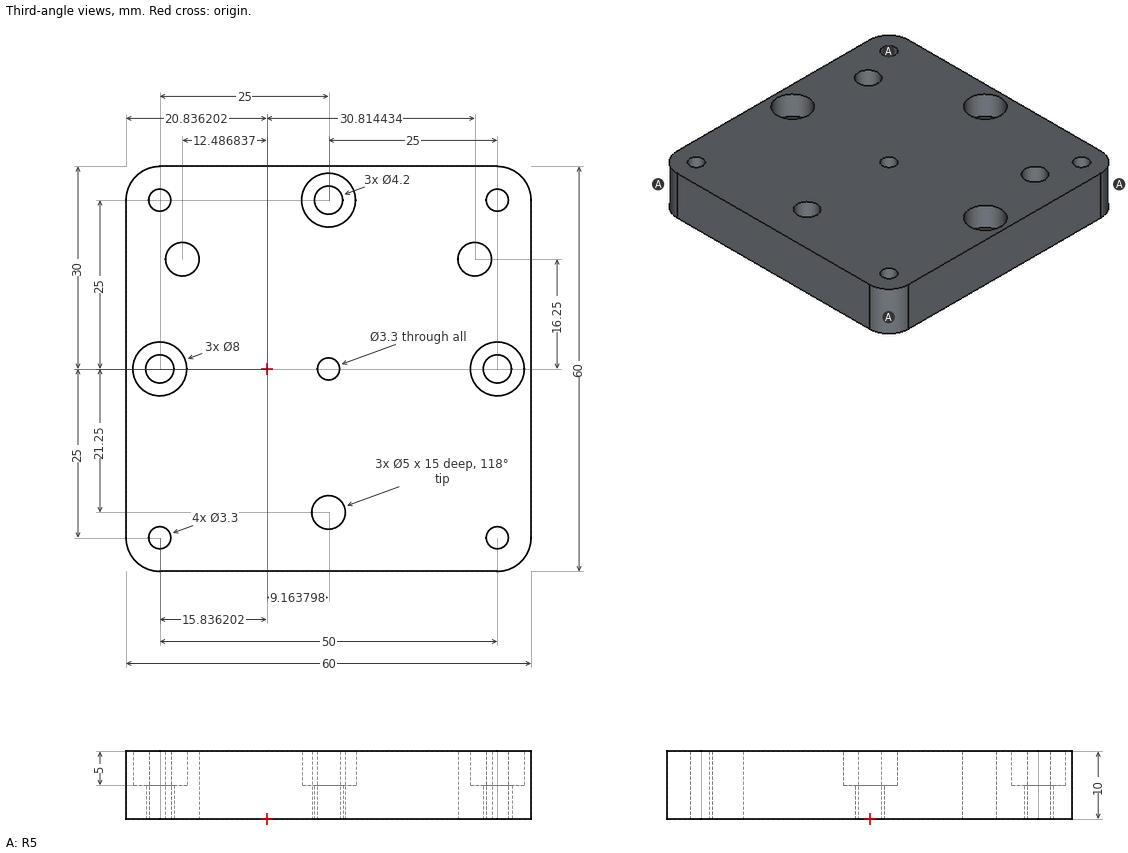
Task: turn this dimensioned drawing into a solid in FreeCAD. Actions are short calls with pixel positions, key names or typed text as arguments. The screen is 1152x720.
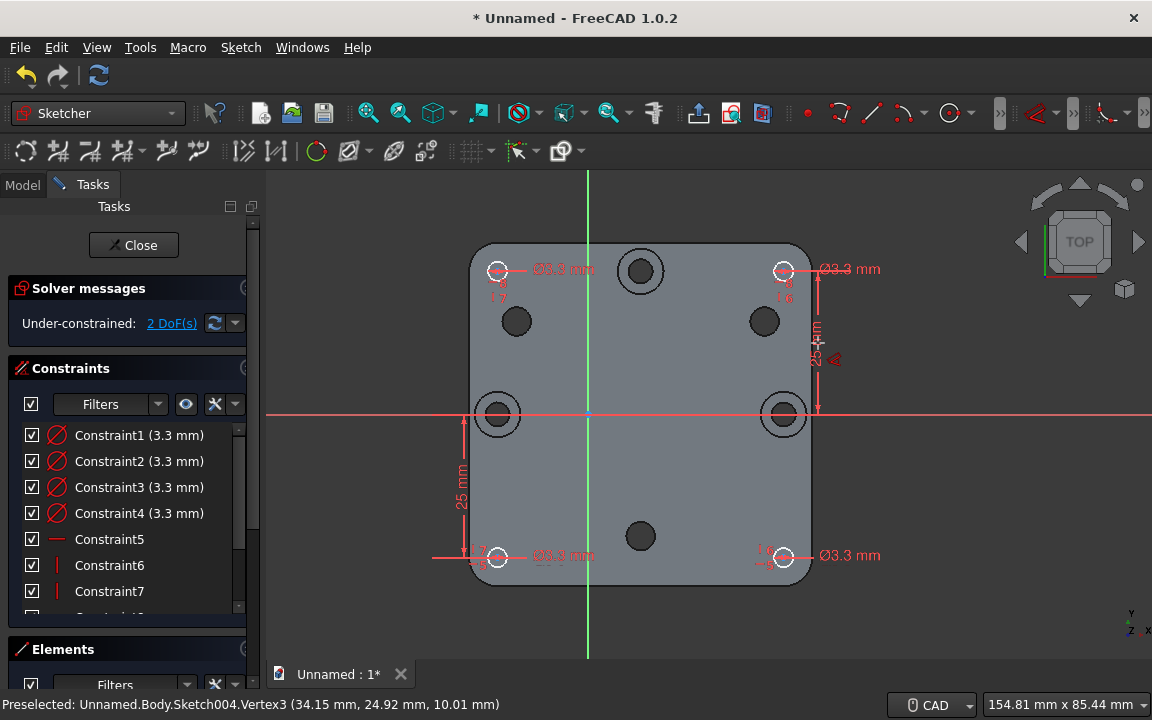
click(498, 558)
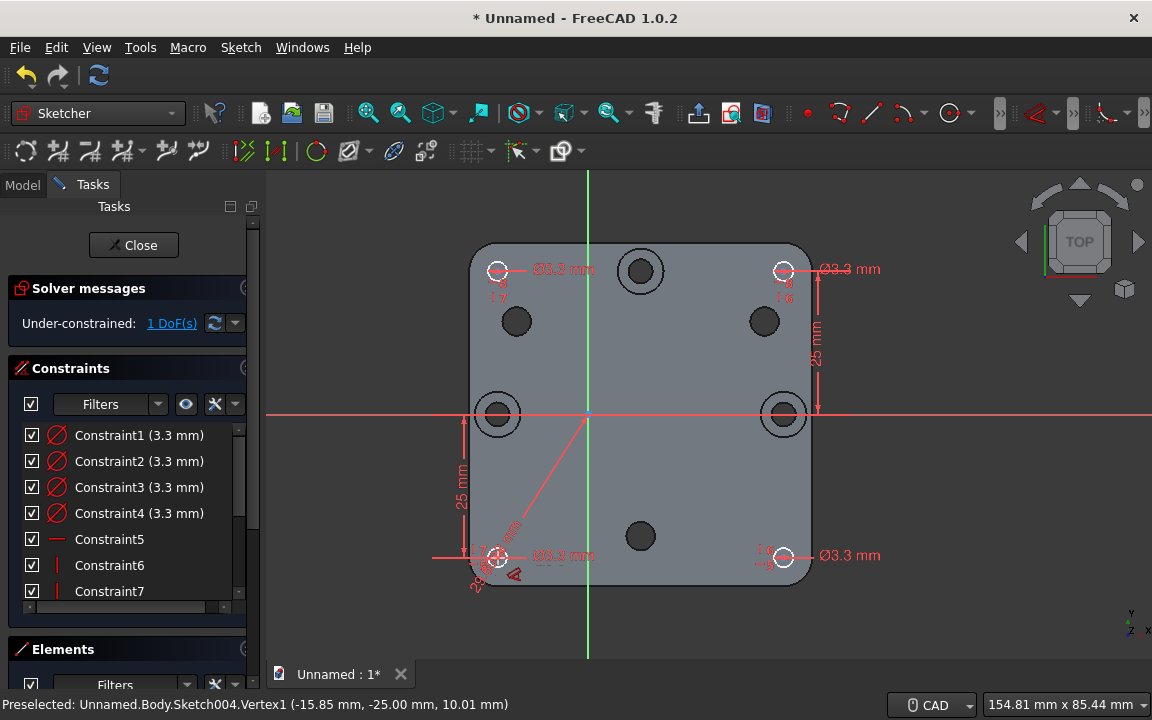
click(784, 558)
click(641, 592)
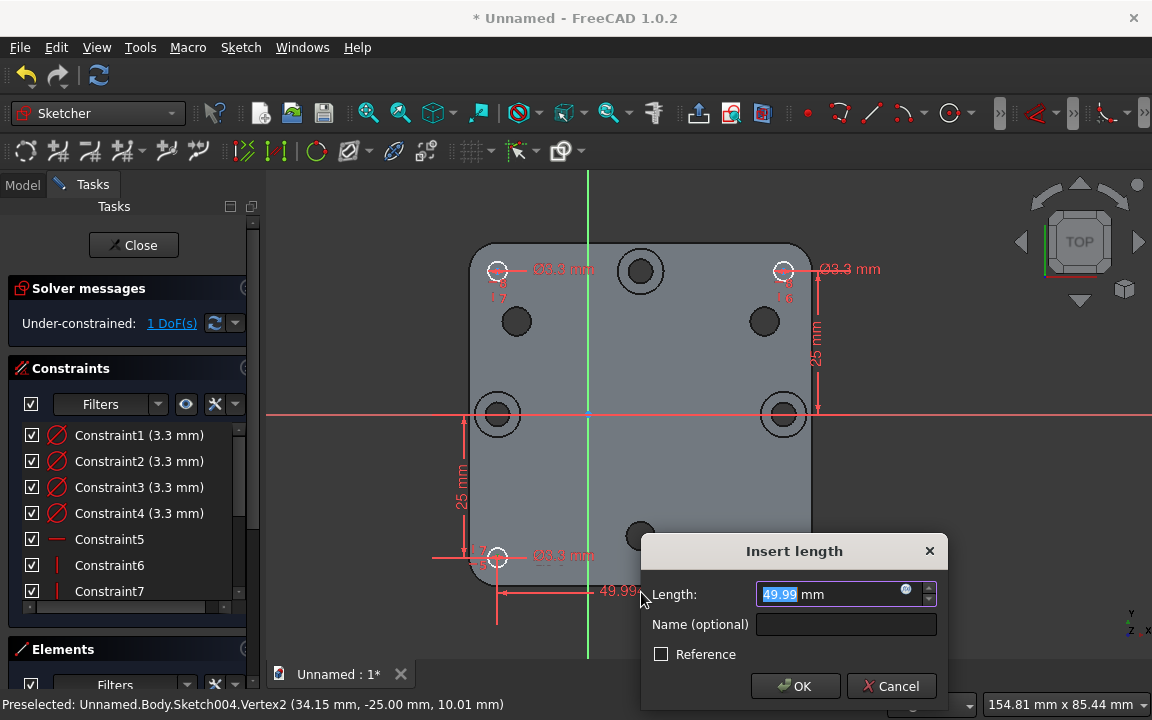
text(50)
key(Return)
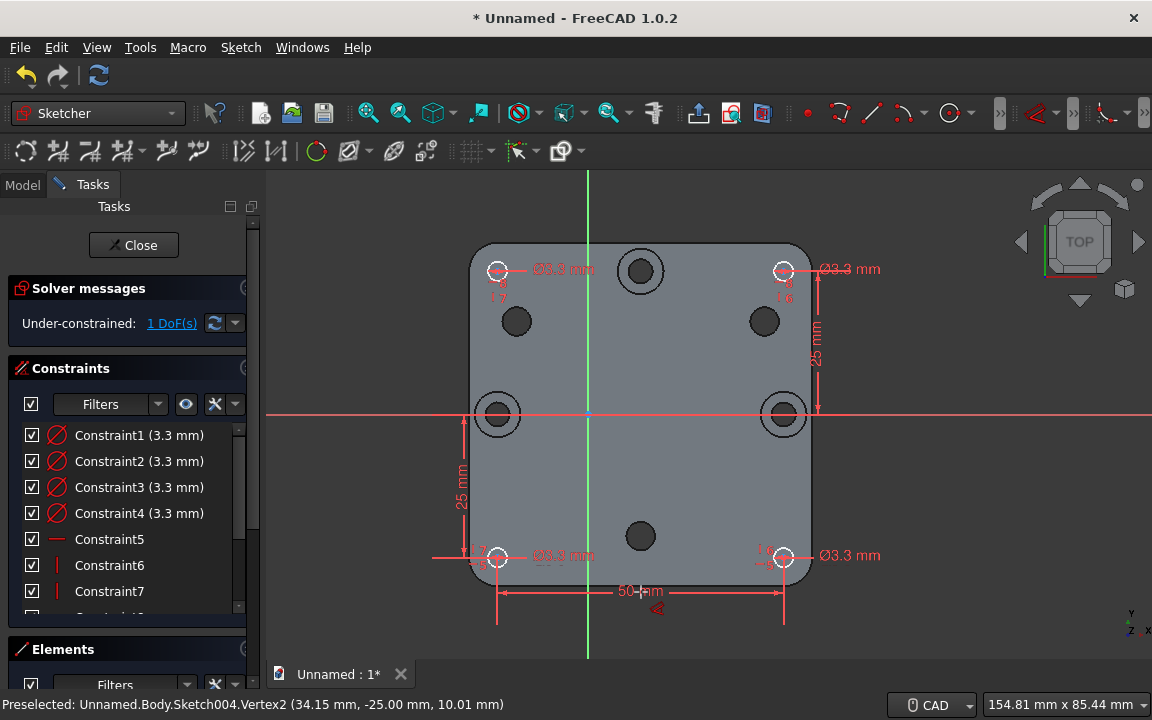
click(497, 558)
click(543, 592)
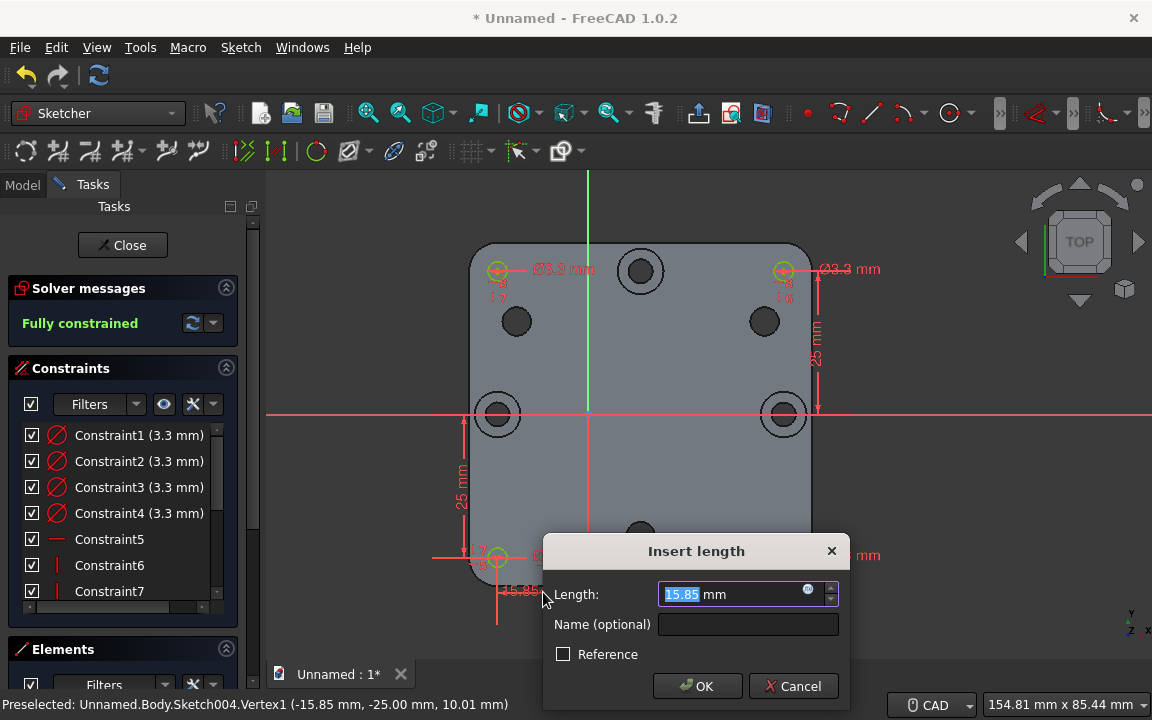
text(15.836202)
key(Return)
key(Escape)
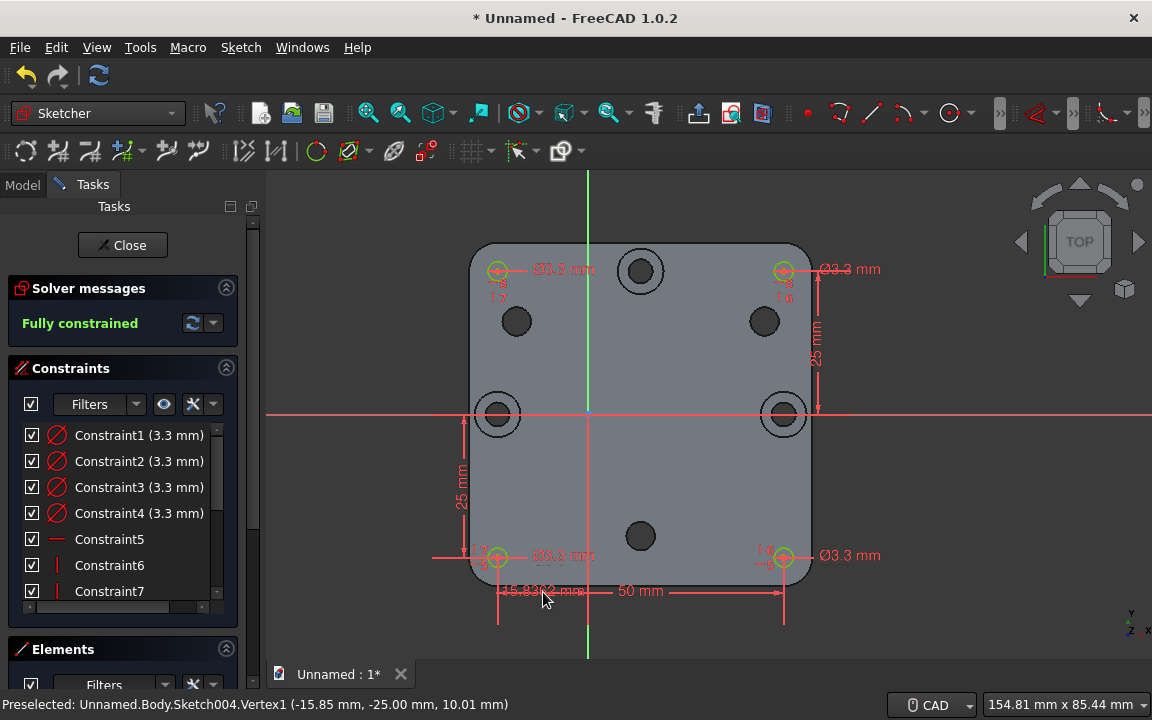
click(123, 245)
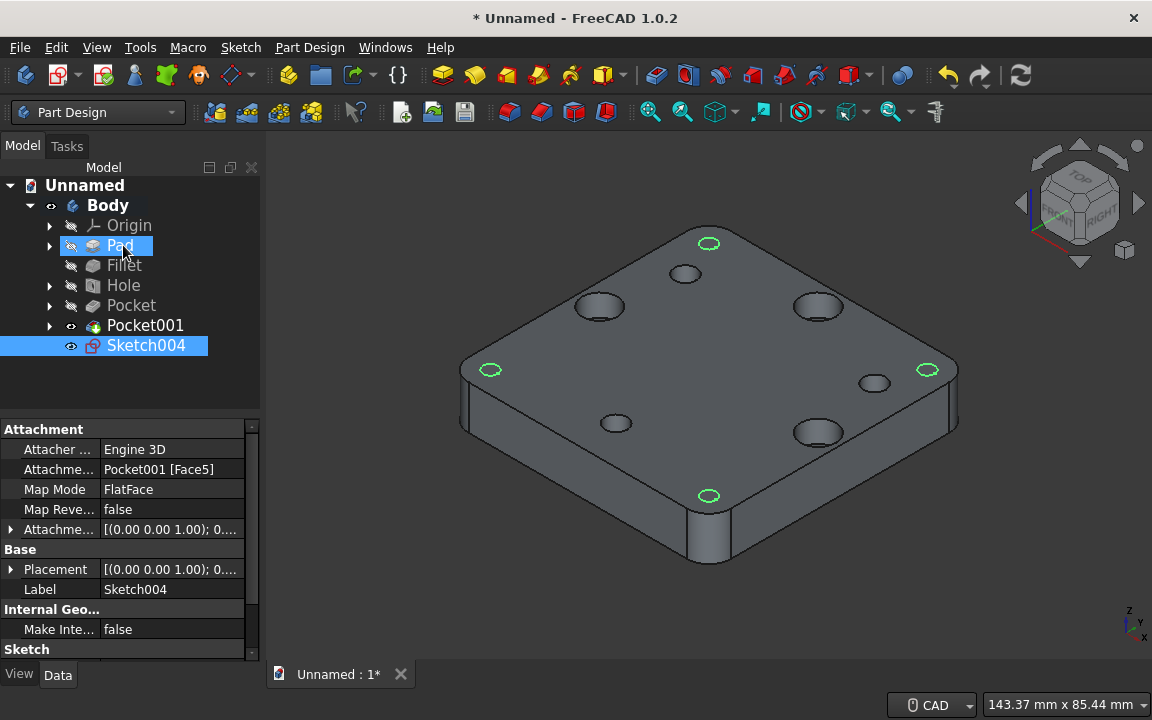
click(658, 76)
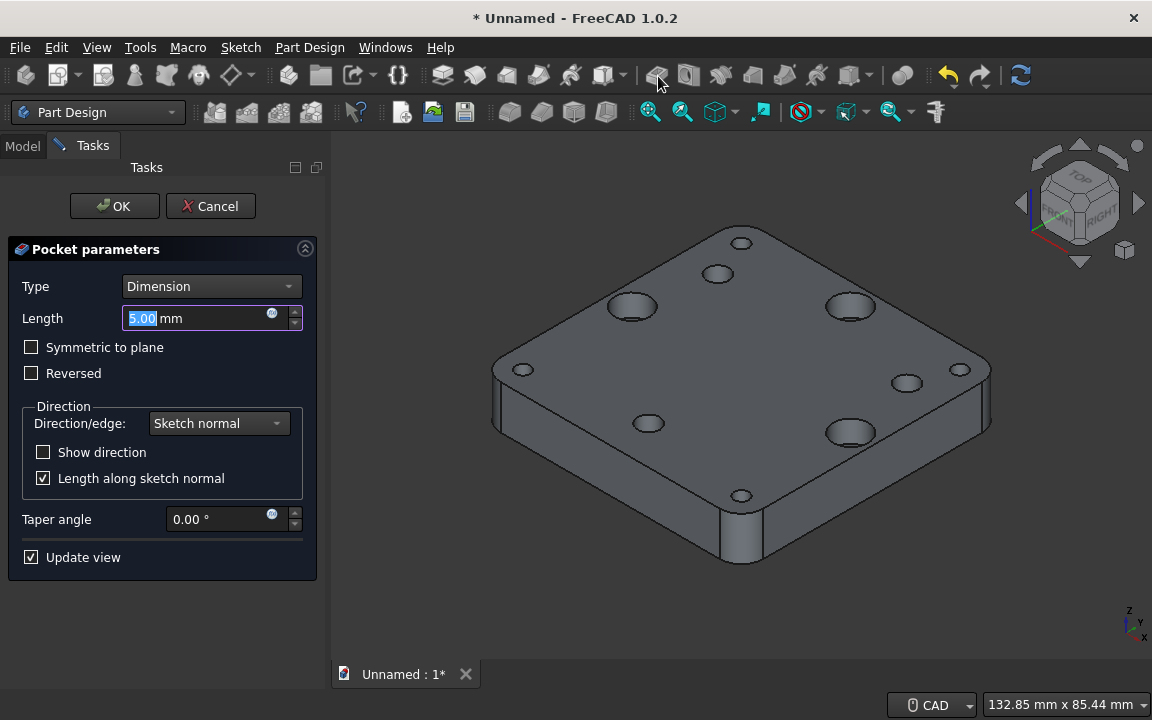
click(212, 286)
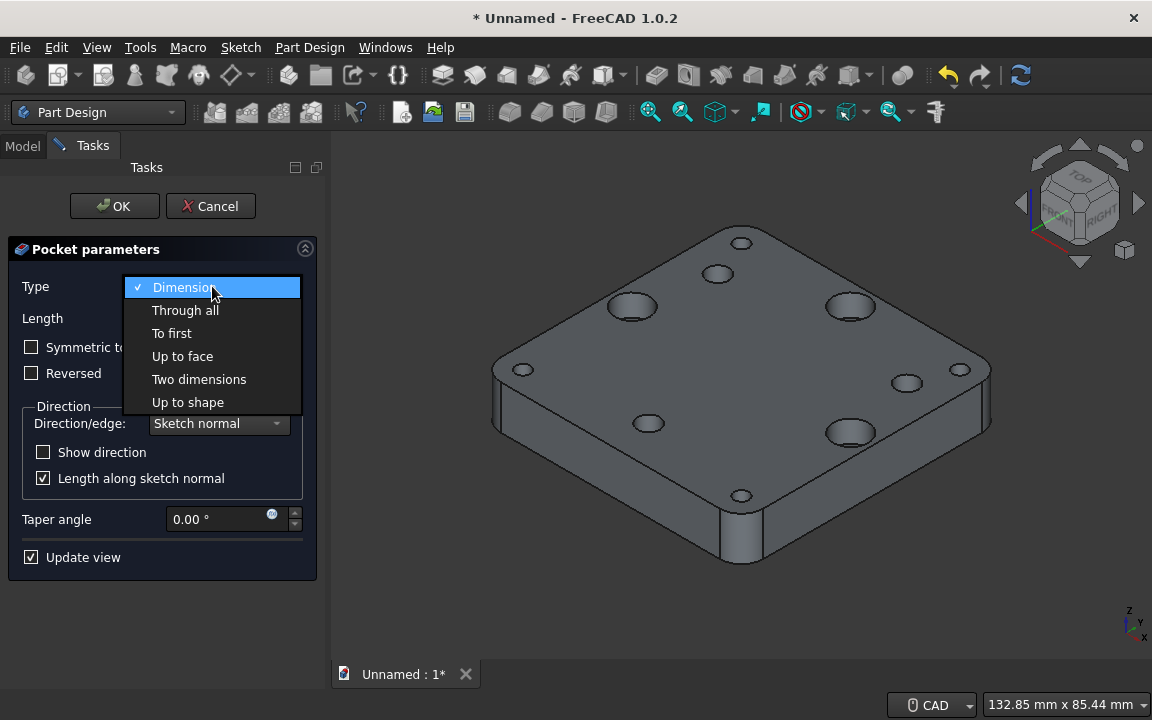
click(212, 310)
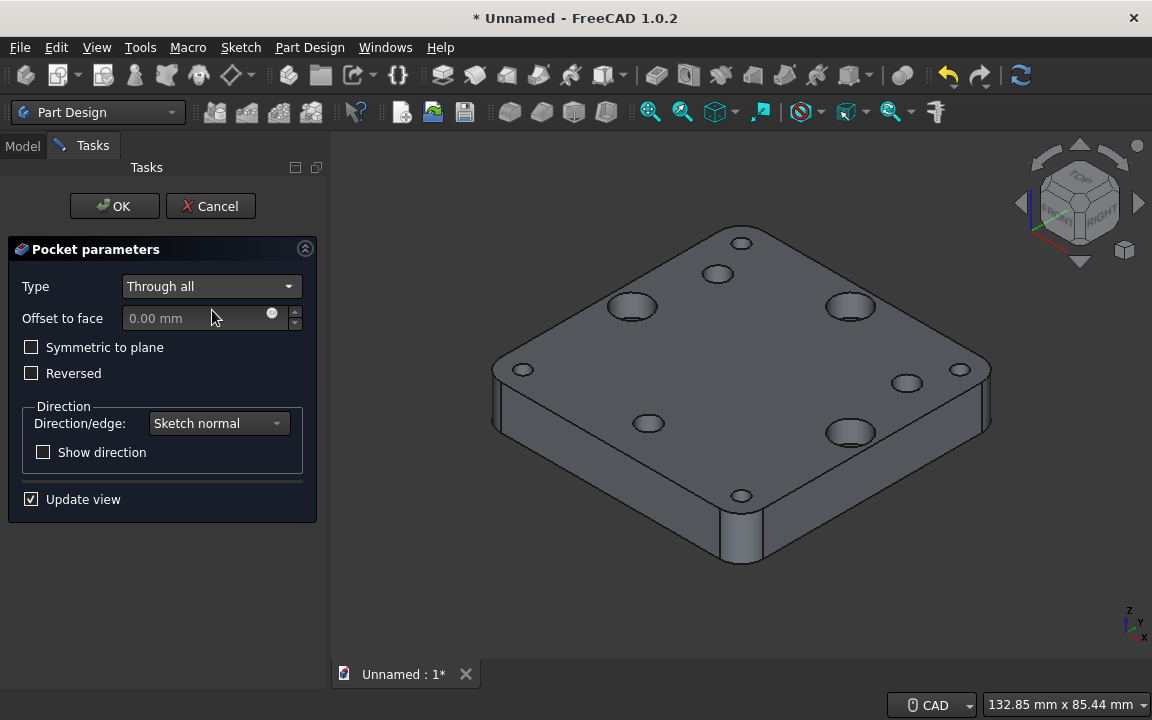
click(115, 206)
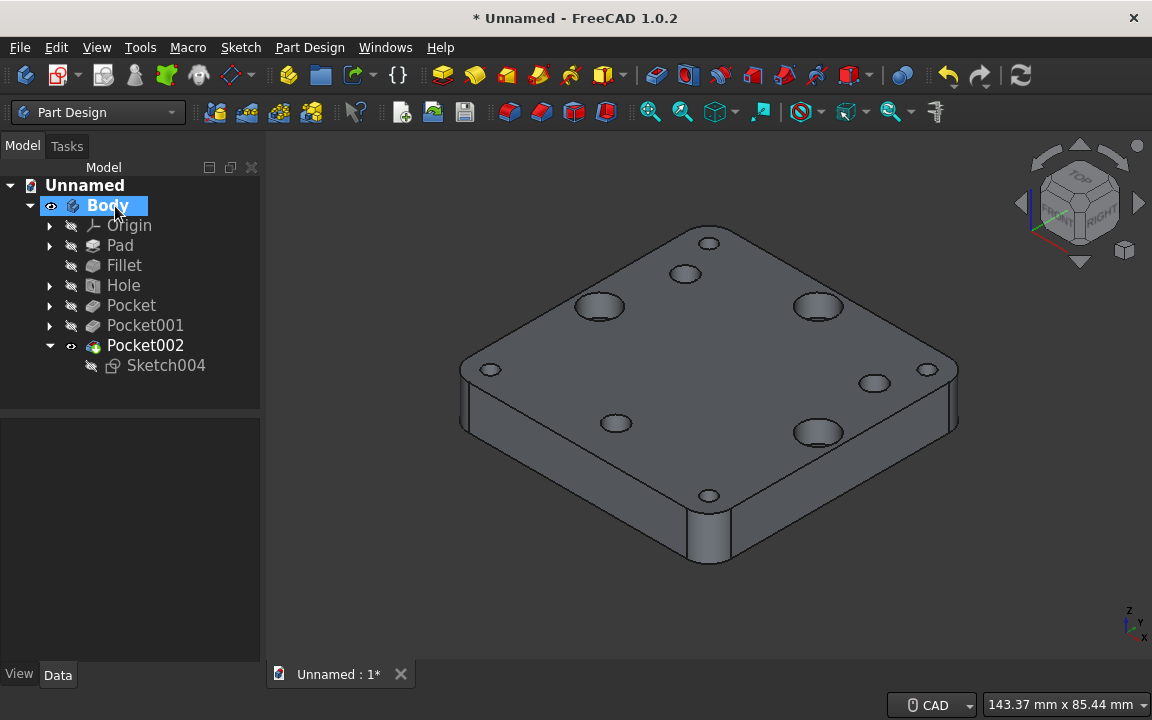
click(709, 369)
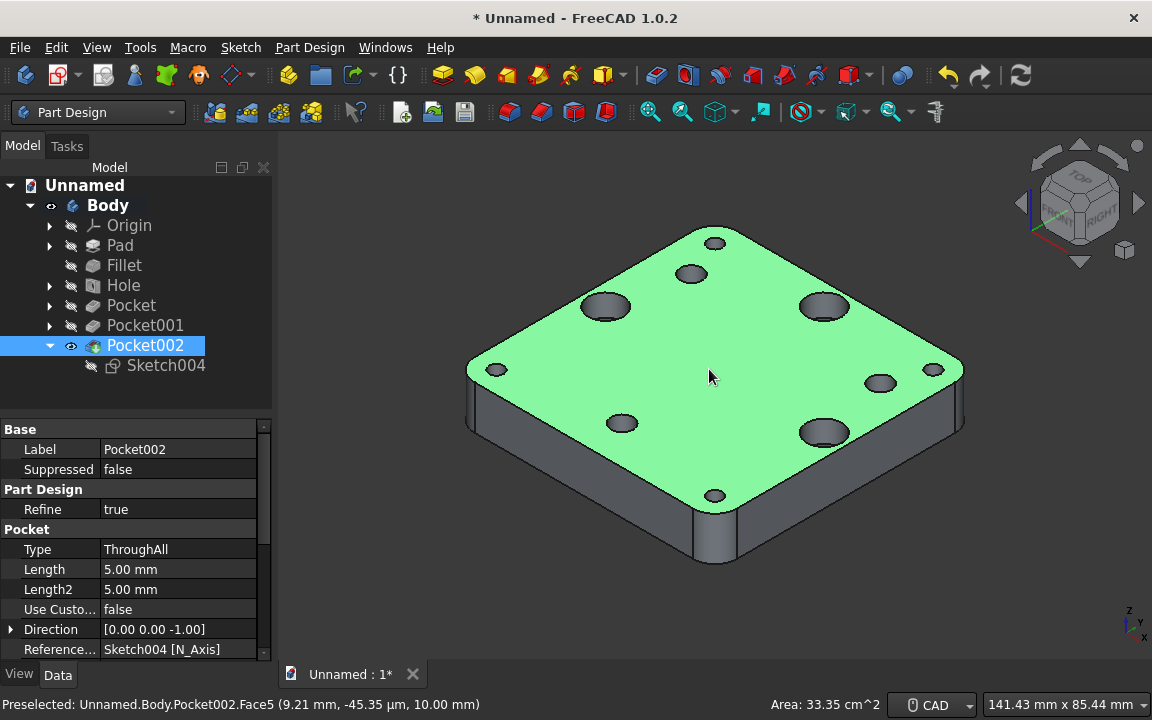
click(58, 76)